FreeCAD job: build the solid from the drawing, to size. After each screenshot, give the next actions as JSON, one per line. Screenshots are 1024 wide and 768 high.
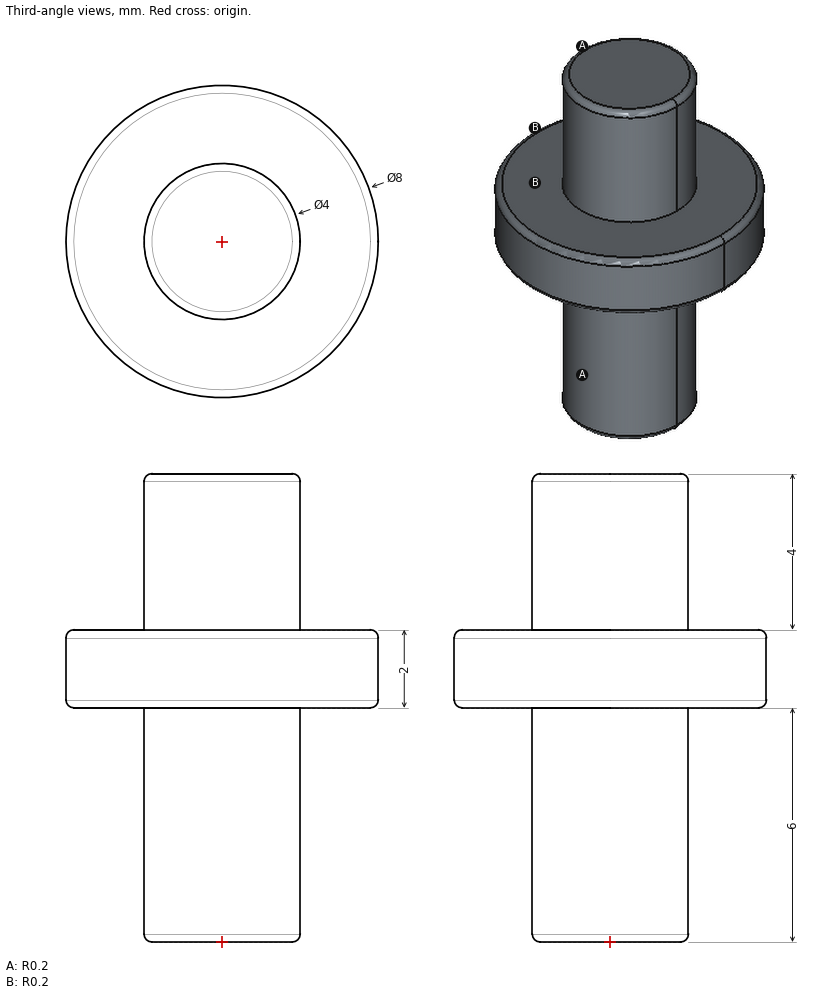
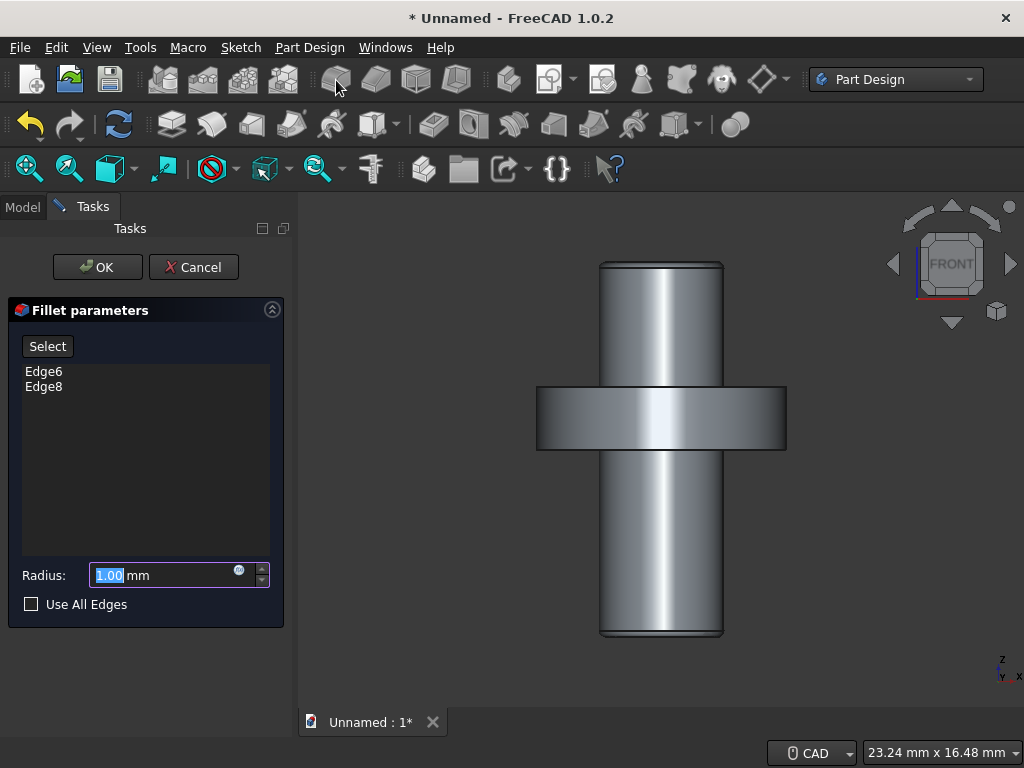
{"action": "type", "text": "0.2"}
{"action": "key", "text": "Tab"}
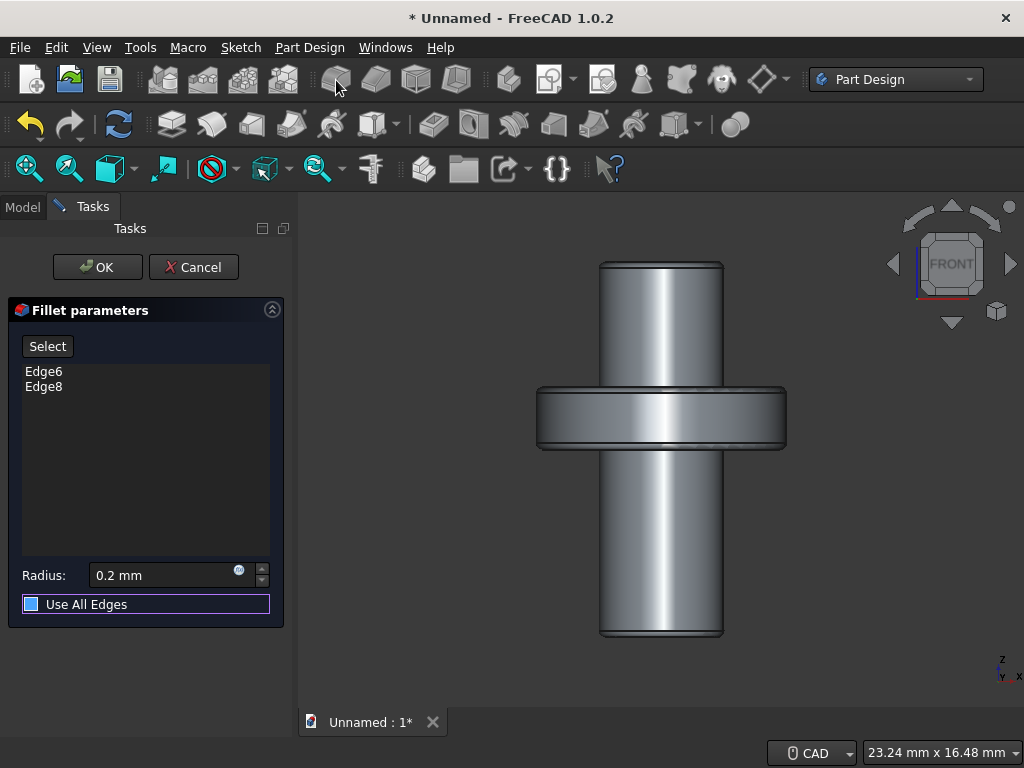
{"action": "left_click", "coordinate": [98, 267]}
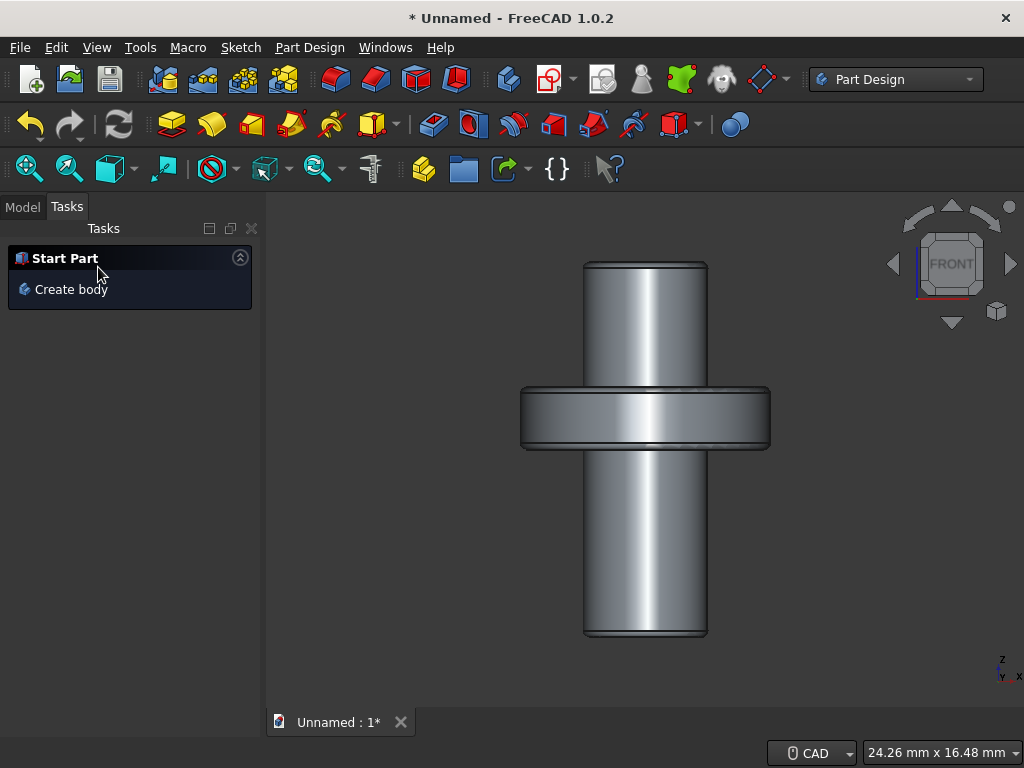
{"action": "key", "text": "0"}